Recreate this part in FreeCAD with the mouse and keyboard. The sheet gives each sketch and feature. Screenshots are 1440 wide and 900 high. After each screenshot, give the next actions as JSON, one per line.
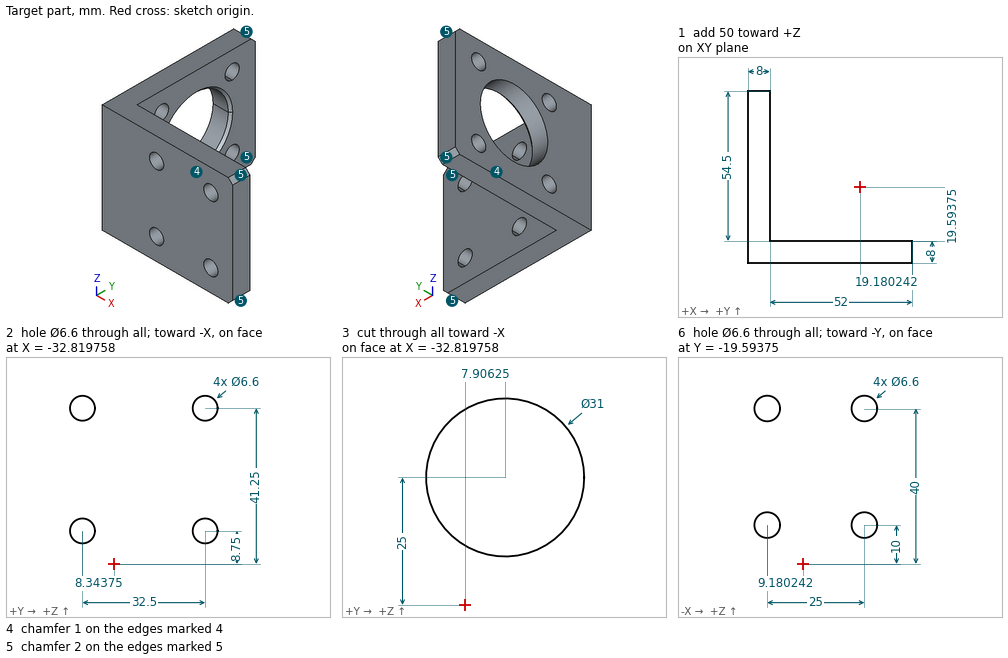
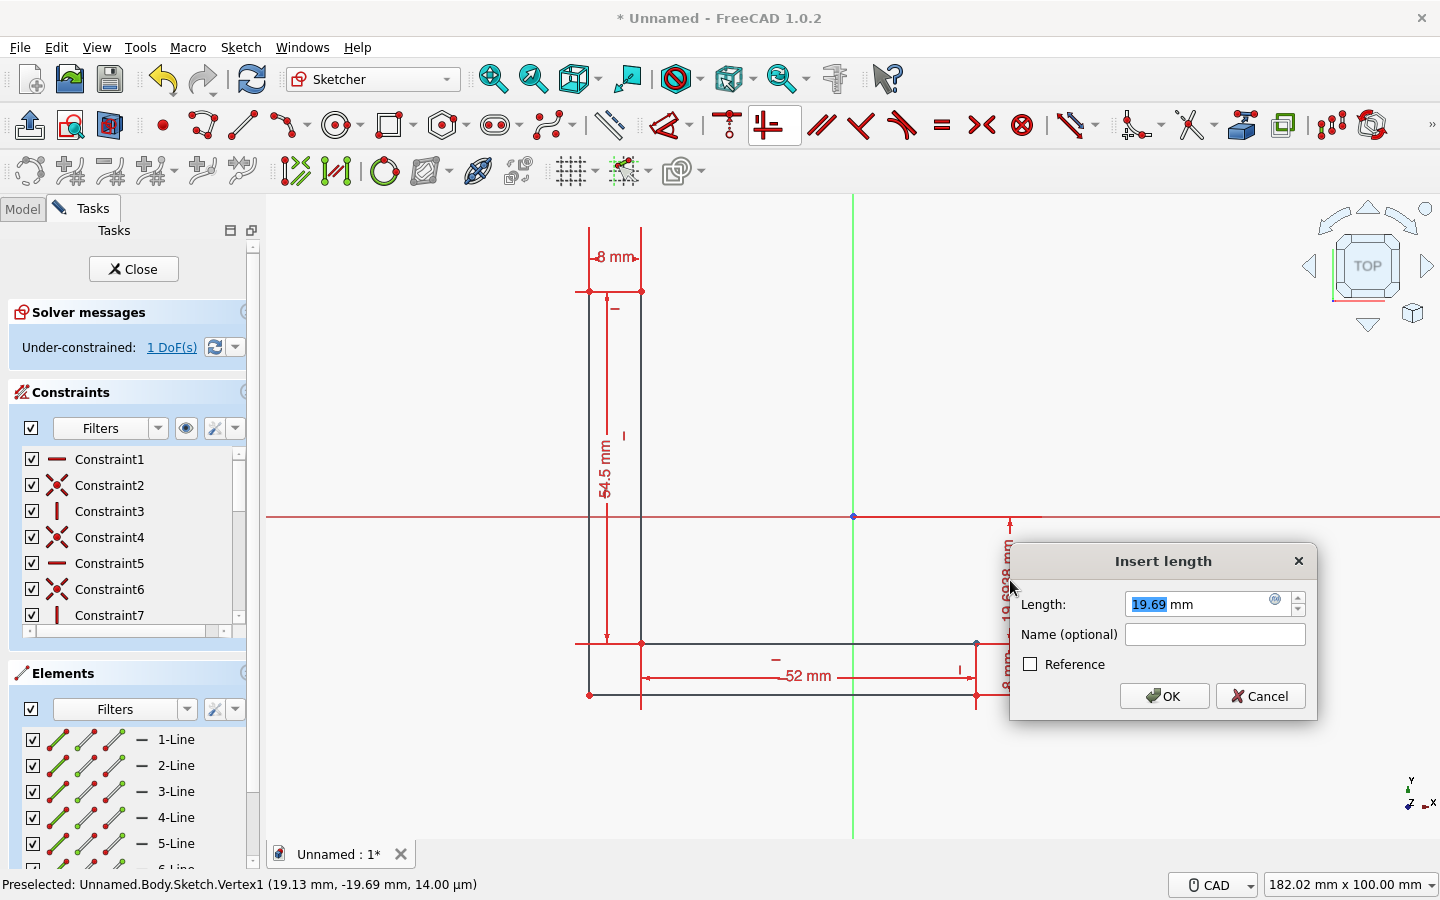
{"action": "type", "text": "19.59375"}
{"action": "key", "text": "Return"}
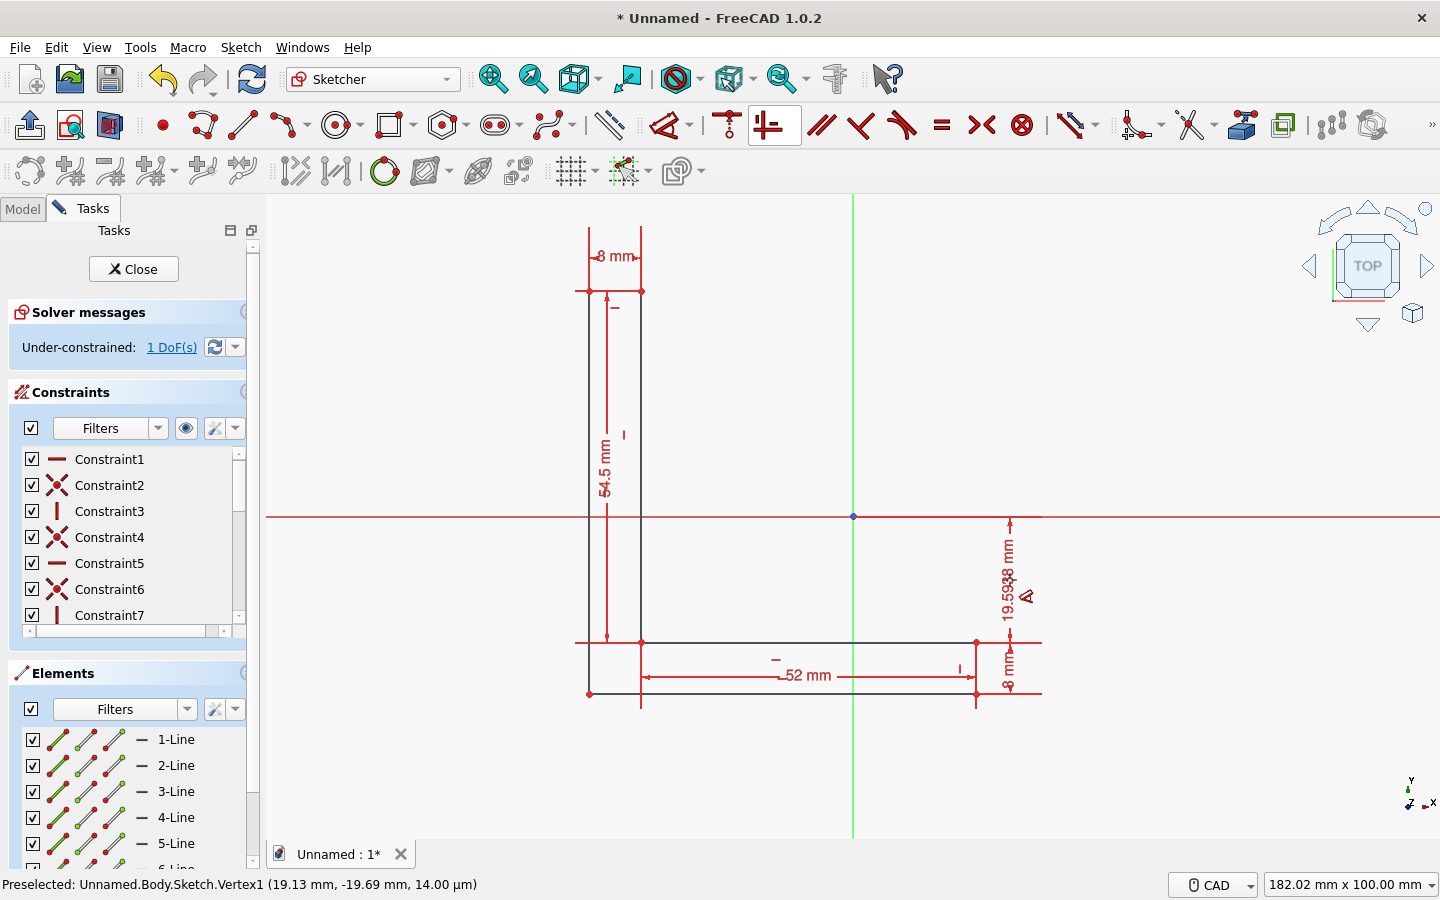
{"action": "left_click", "coordinate": [976, 643]}
{"action": "left_click", "coordinate": [915, 677]}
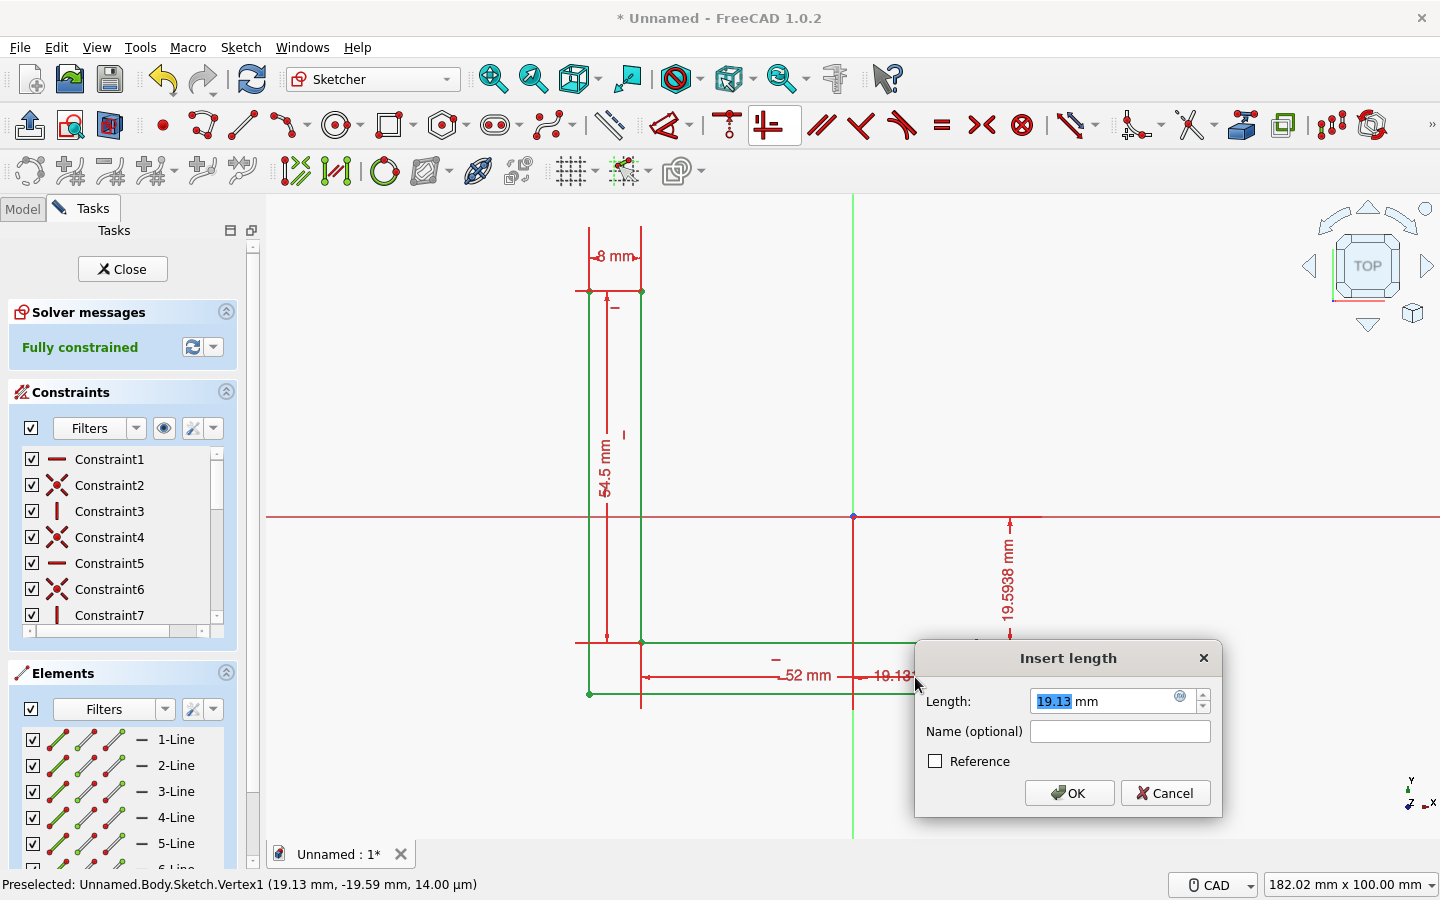
{"action": "type", "text": "19.180242"}
{"action": "key", "text": "Return"}
{"action": "key", "text": "Escape"}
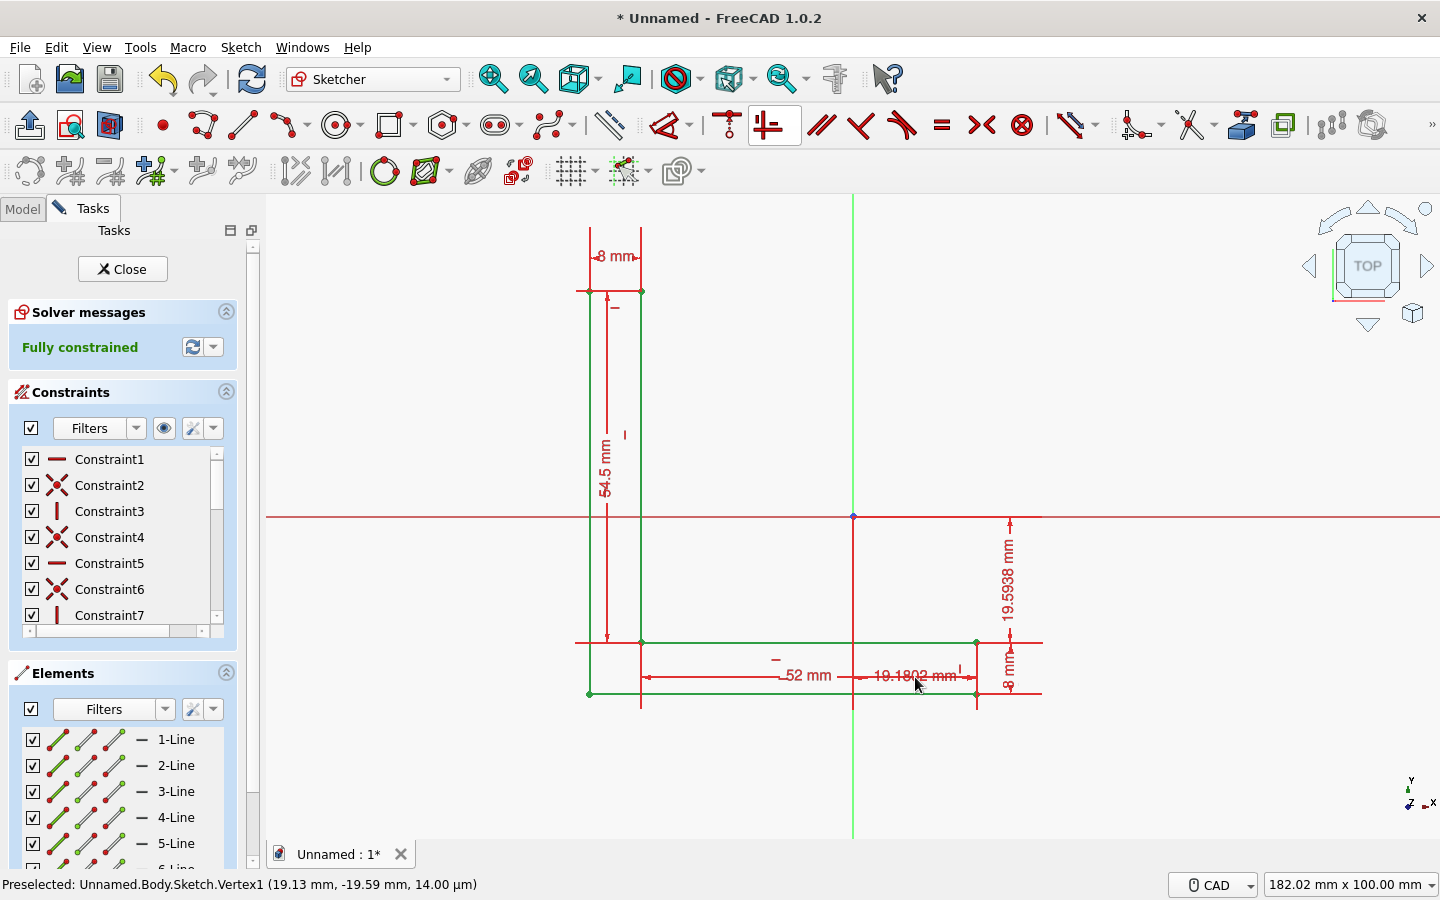
{"action": "left_click", "coordinate": [123, 269]}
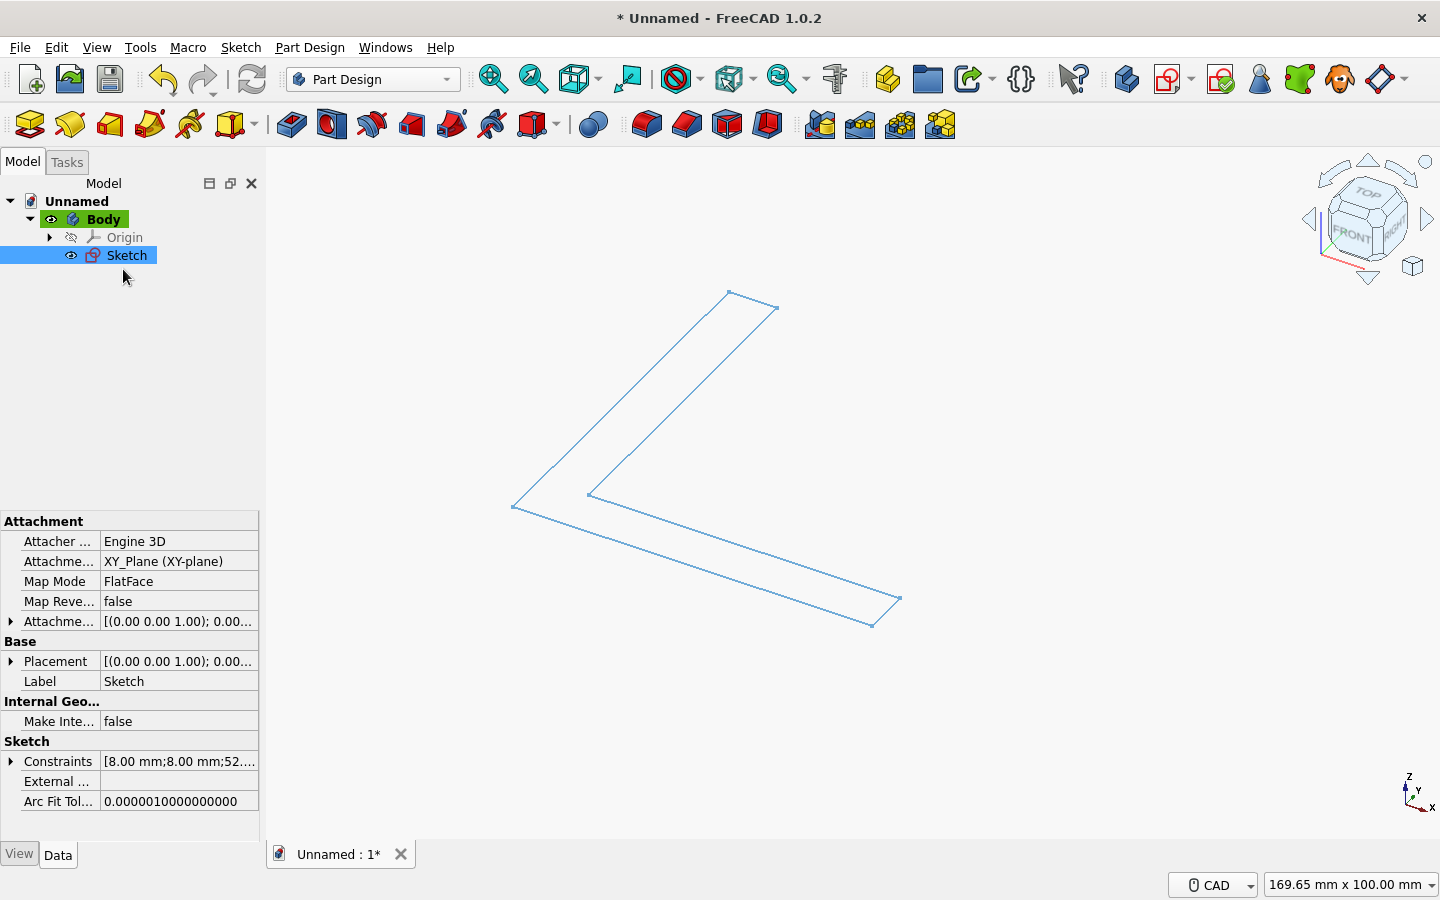
{"action": "left_click", "coordinate": [30, 124]}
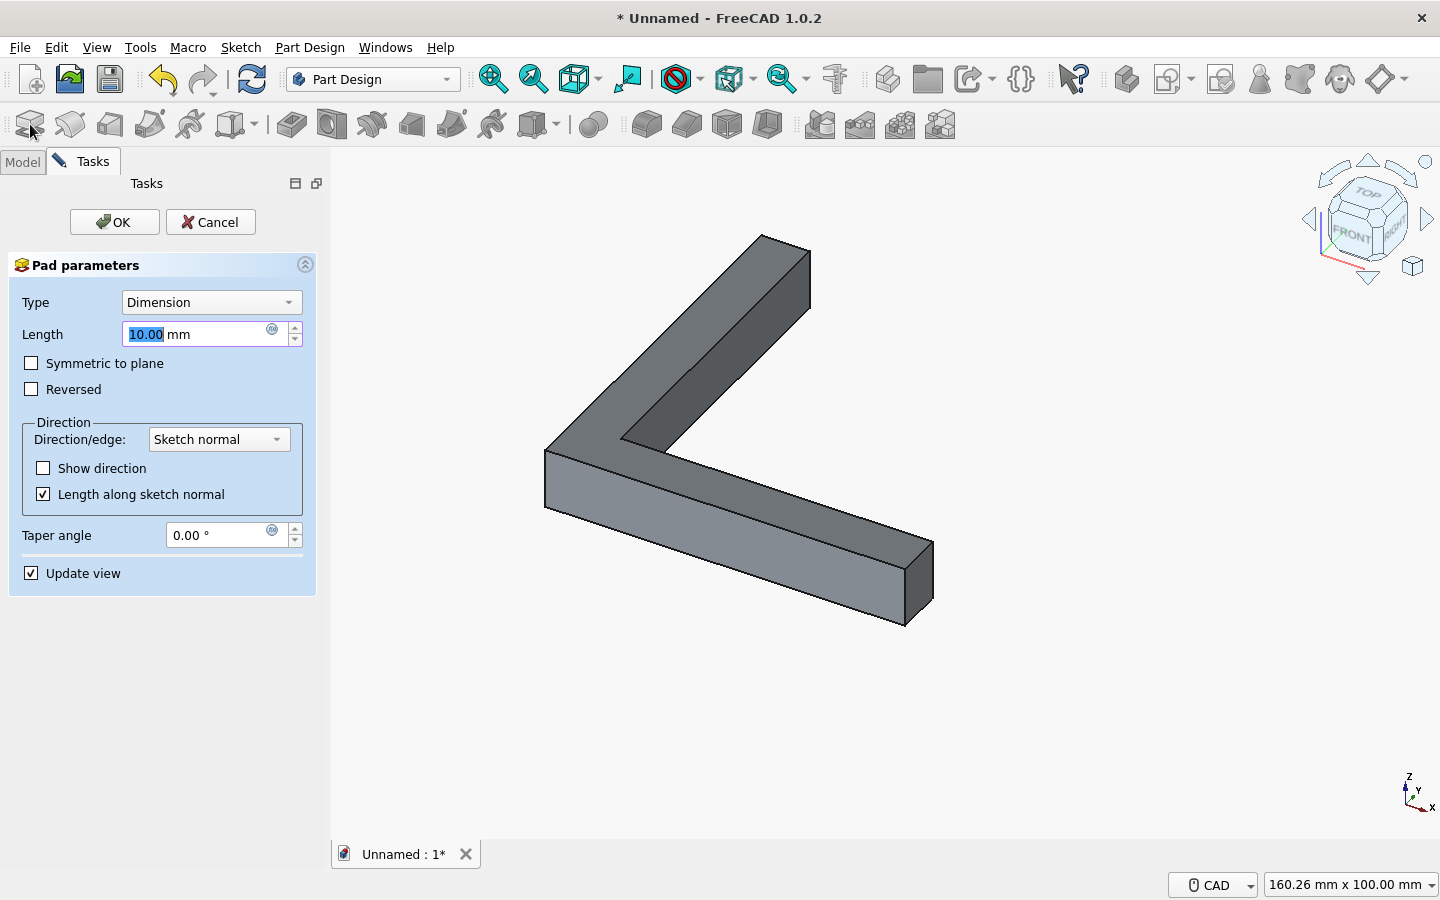
{"action": "type", "text": "50"}
{"action": "key", "text": "Tab"}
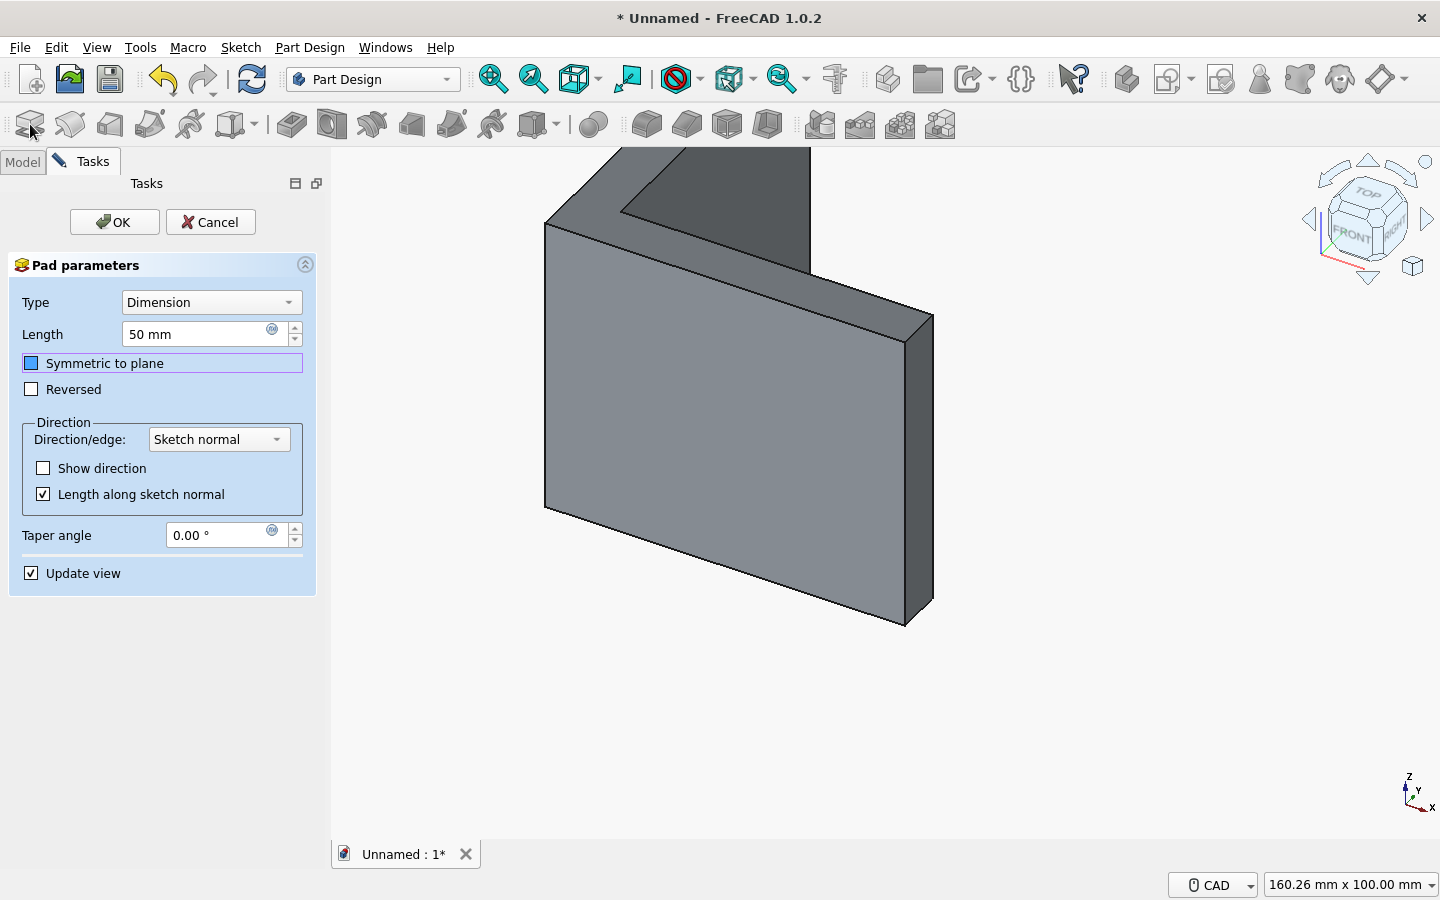
{"action": "left_click", "coordinate": [115, 222]}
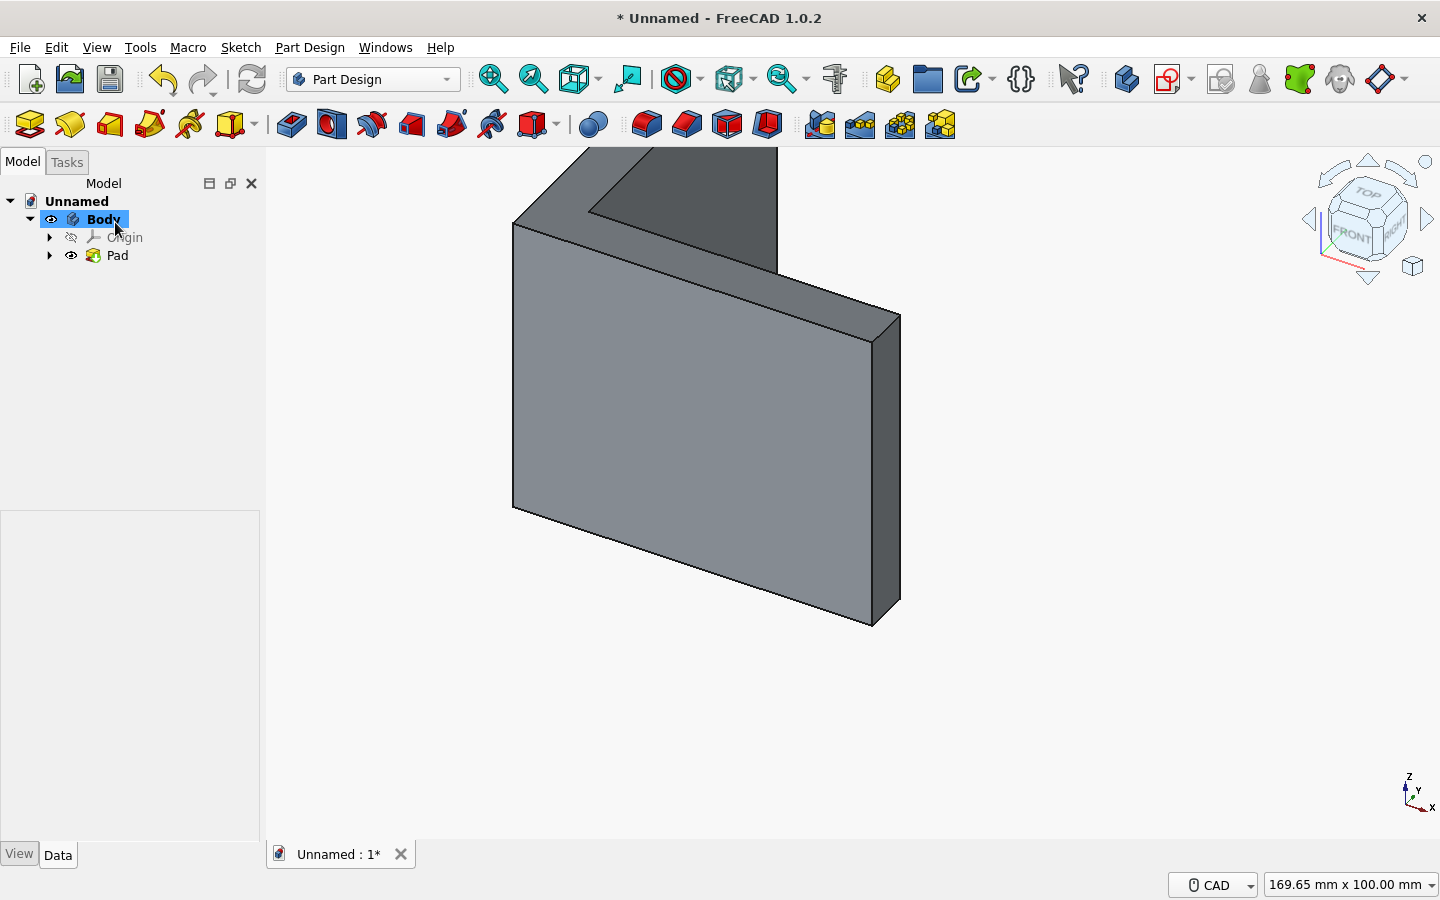
{"action": "left_click", "coordinate": [494, 80]}